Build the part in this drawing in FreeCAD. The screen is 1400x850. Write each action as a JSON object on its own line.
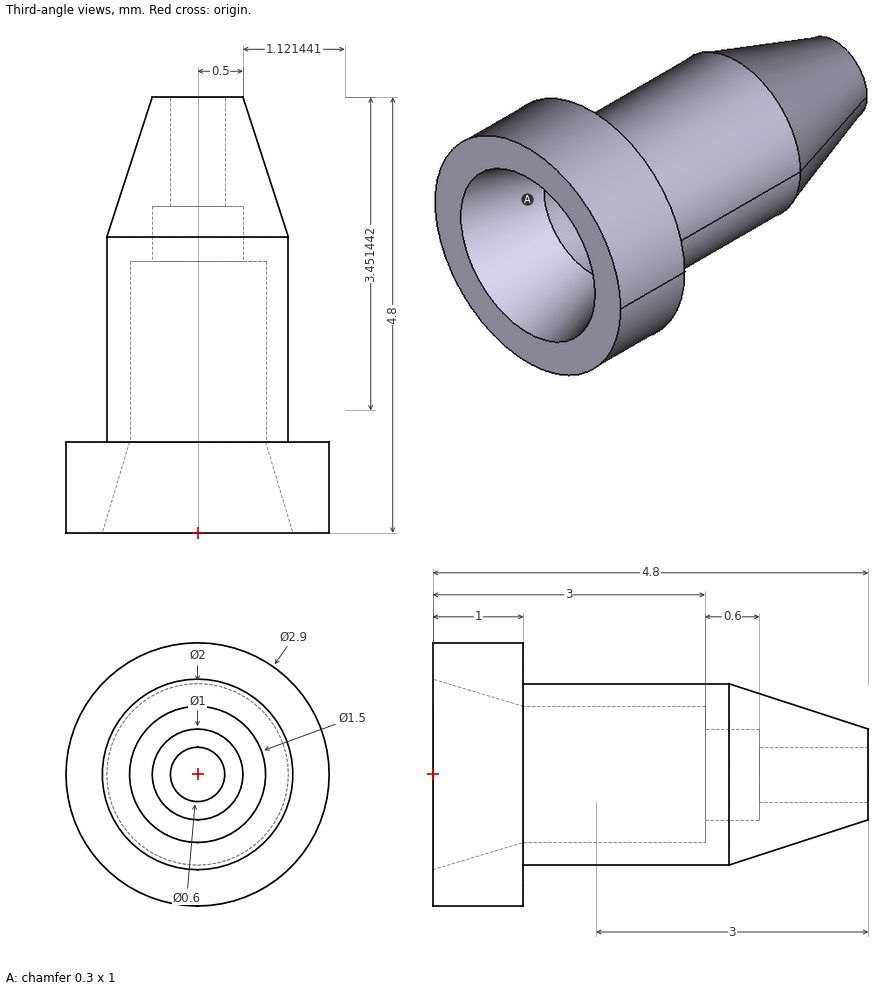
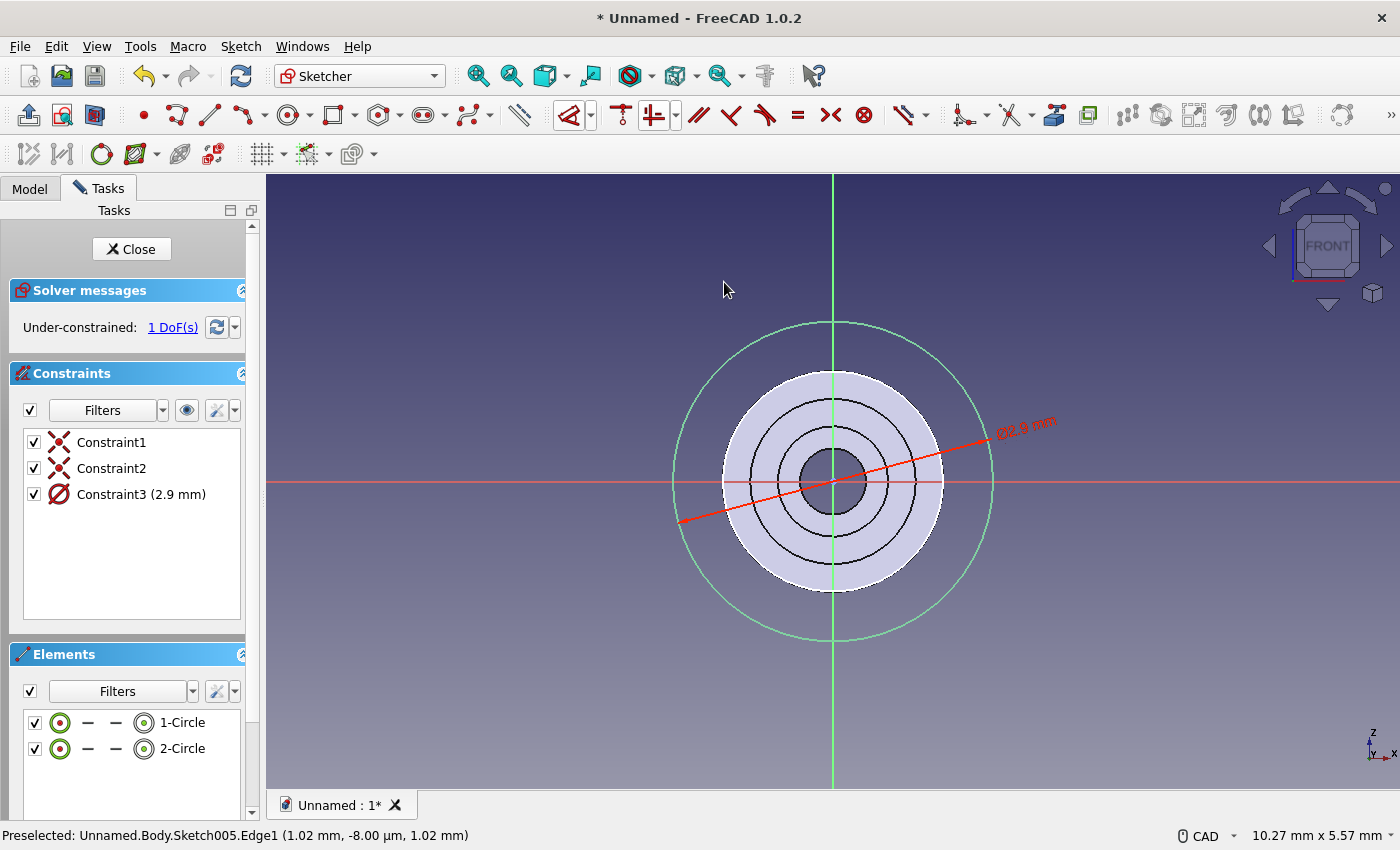
{"action": "left_click", "coordinate": [911, 404]}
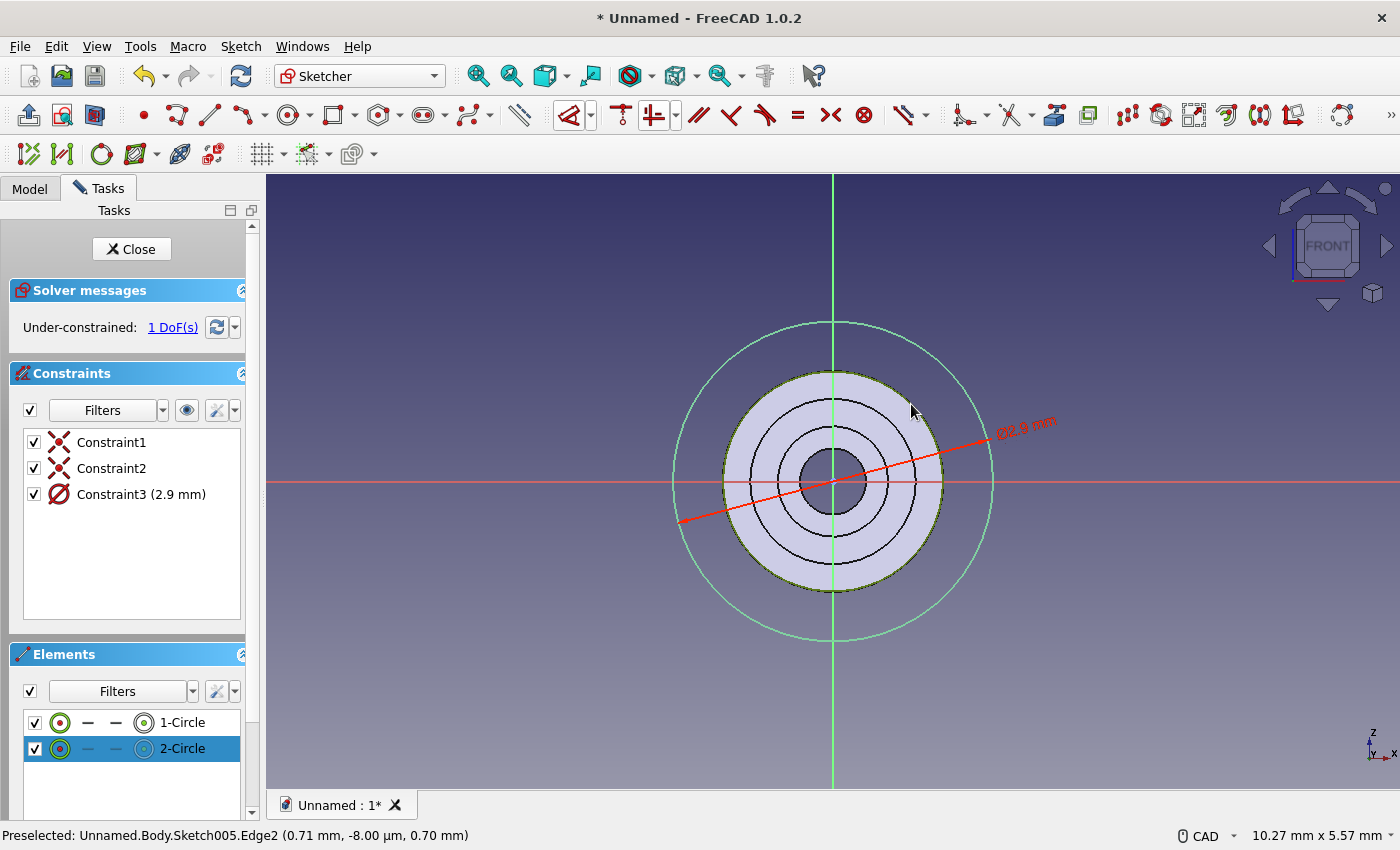
{"action": "key", "text": "k o"}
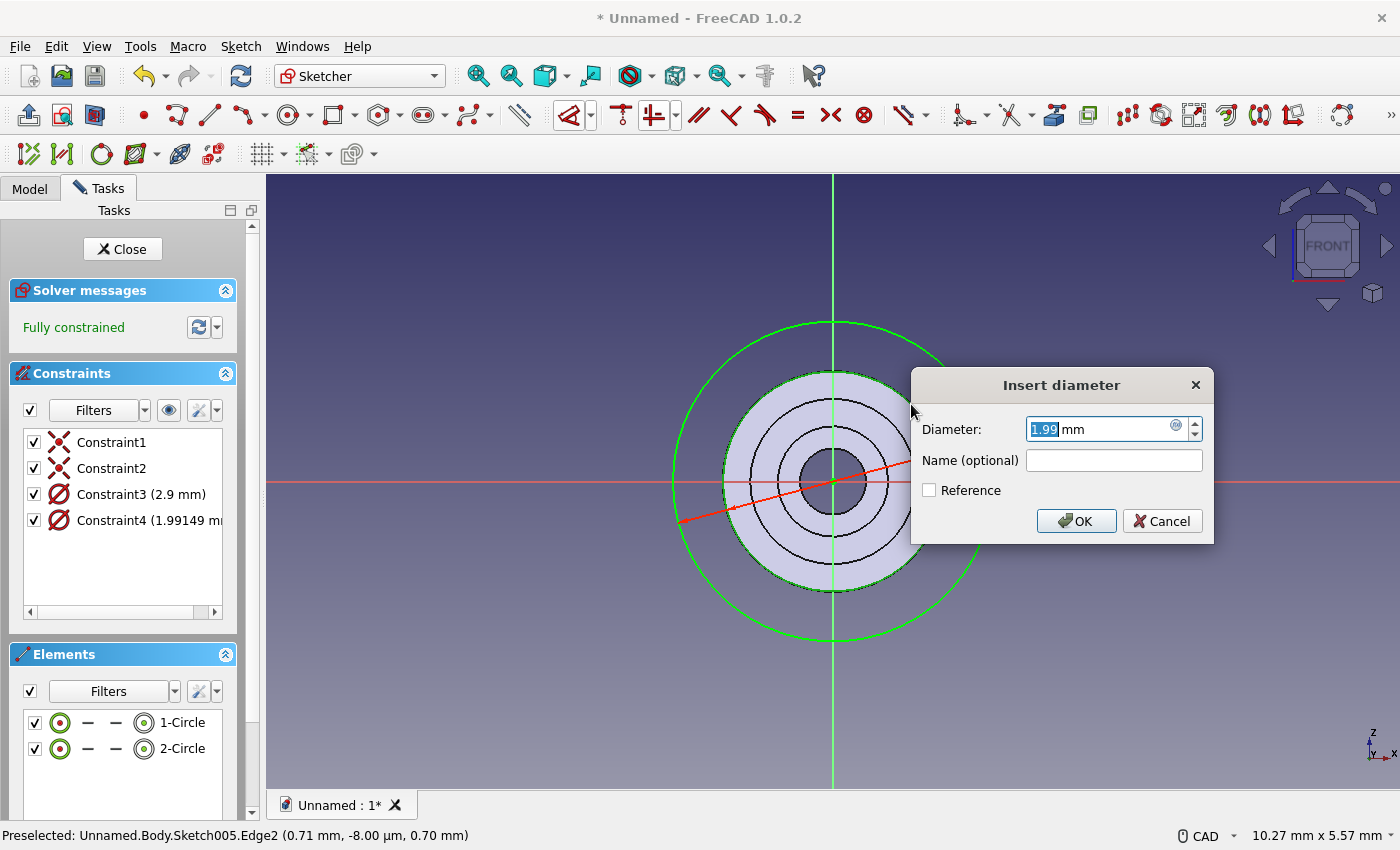
{"action": "type", "text": "2"}
{"action": "key", "text": "Return"}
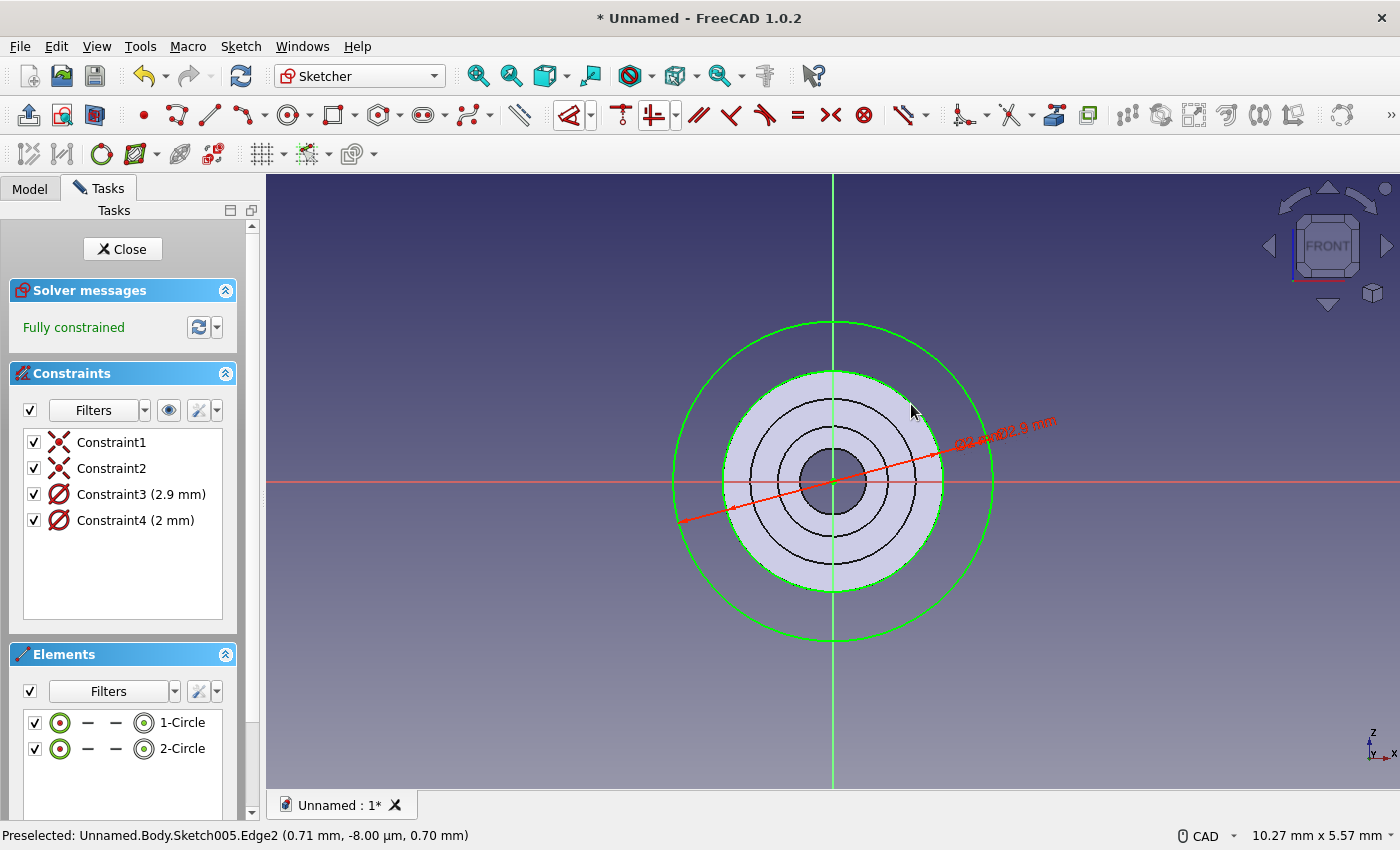
{"action": "left_click", "coordinate": [123, 249]}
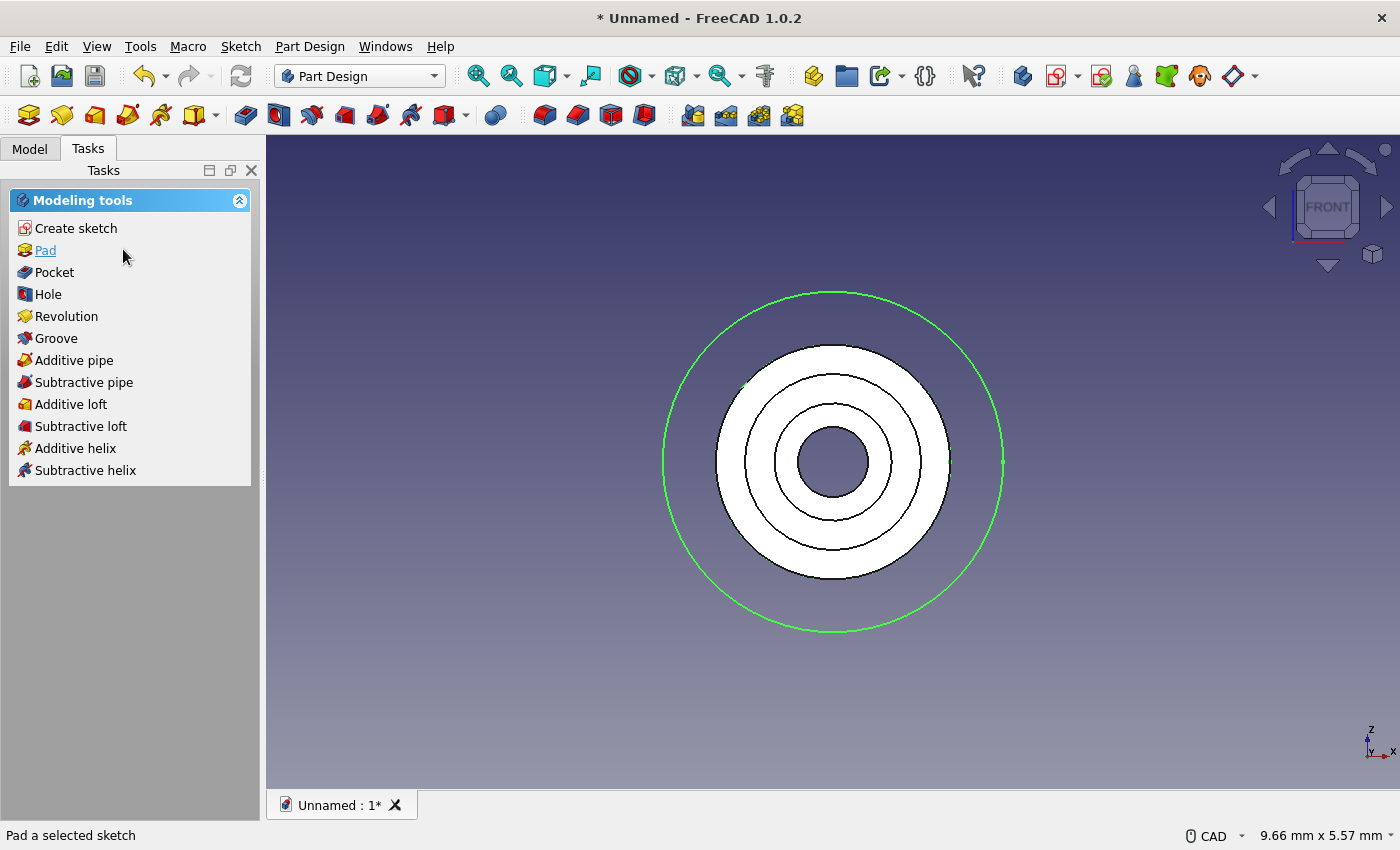
{"action": "left_click", "coordinate": [29, 116]}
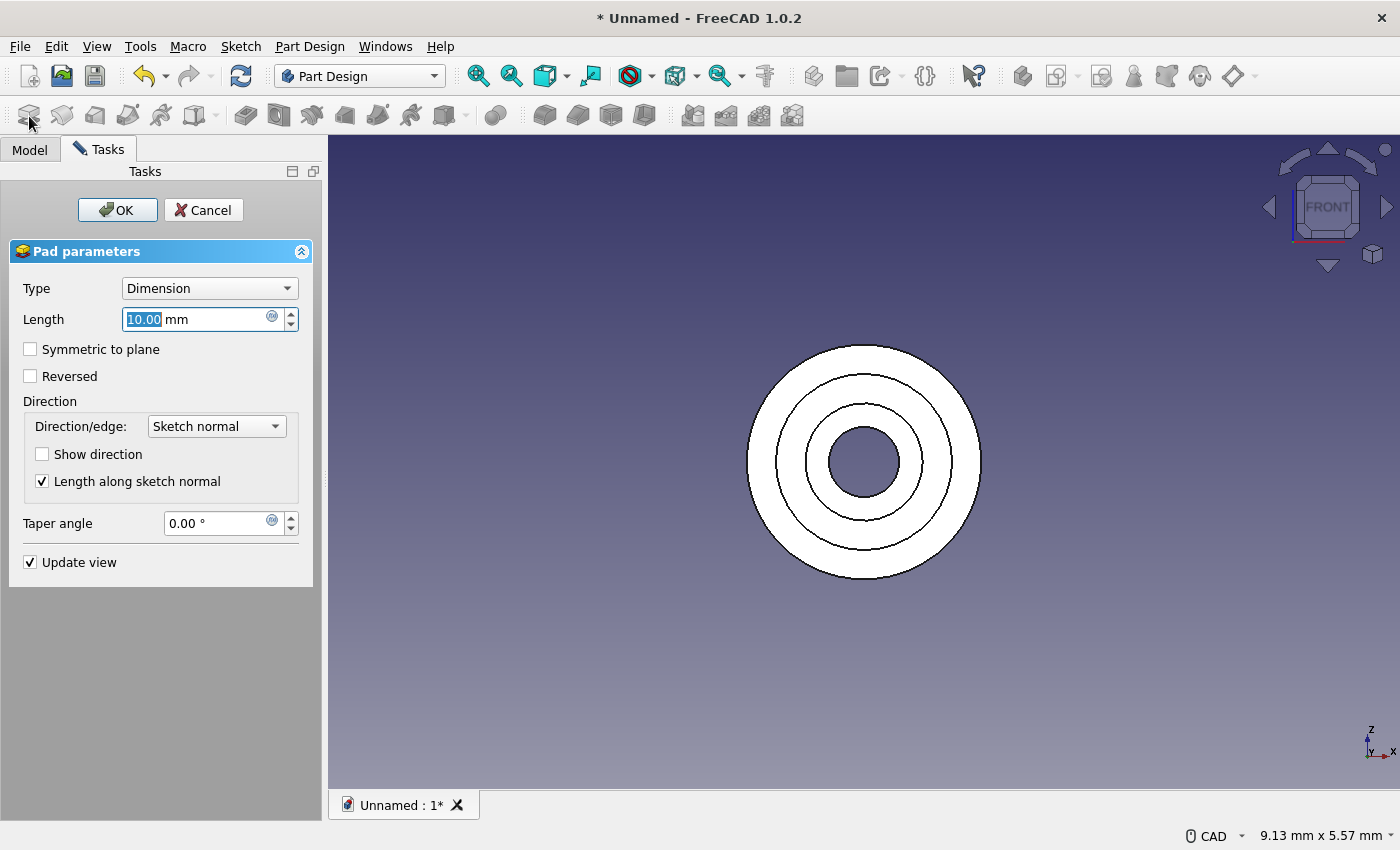
{"action": "type", "text": "1"}
{"action": "key", "text": "Tab"}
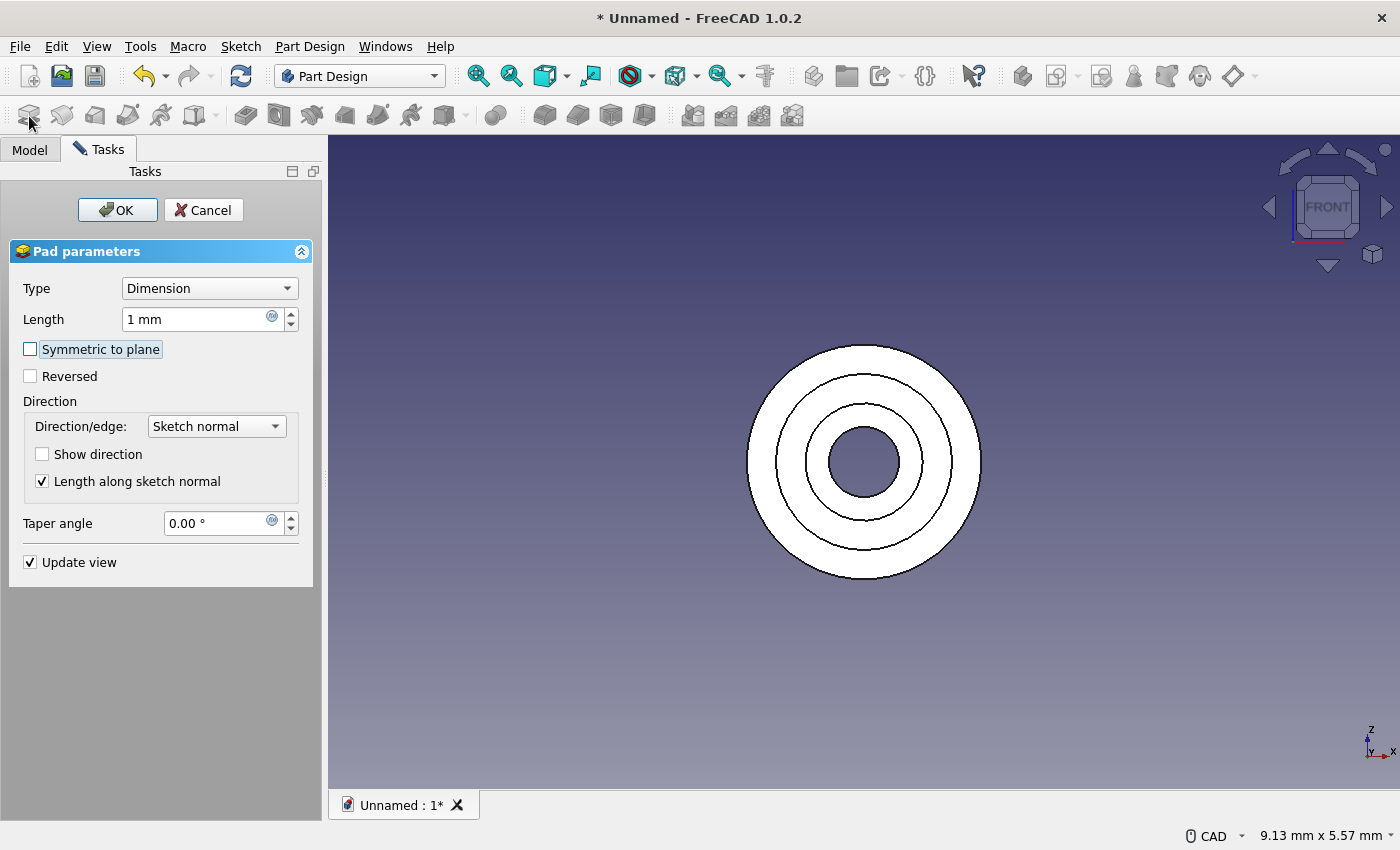
{"action": "left_click", "coordinate": [31, 376]}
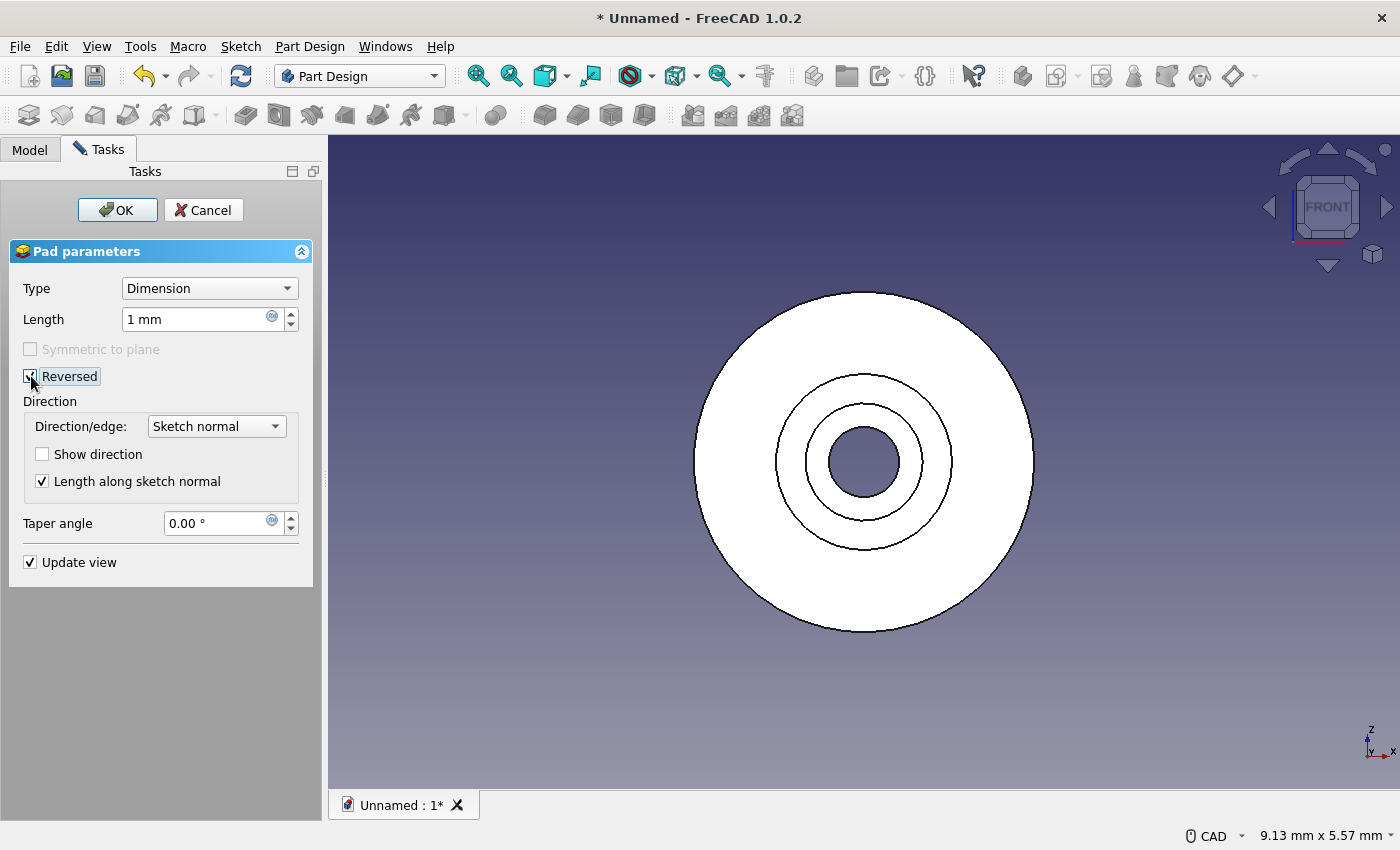
{"action": "left_click", "coordinate": [118, 210]}